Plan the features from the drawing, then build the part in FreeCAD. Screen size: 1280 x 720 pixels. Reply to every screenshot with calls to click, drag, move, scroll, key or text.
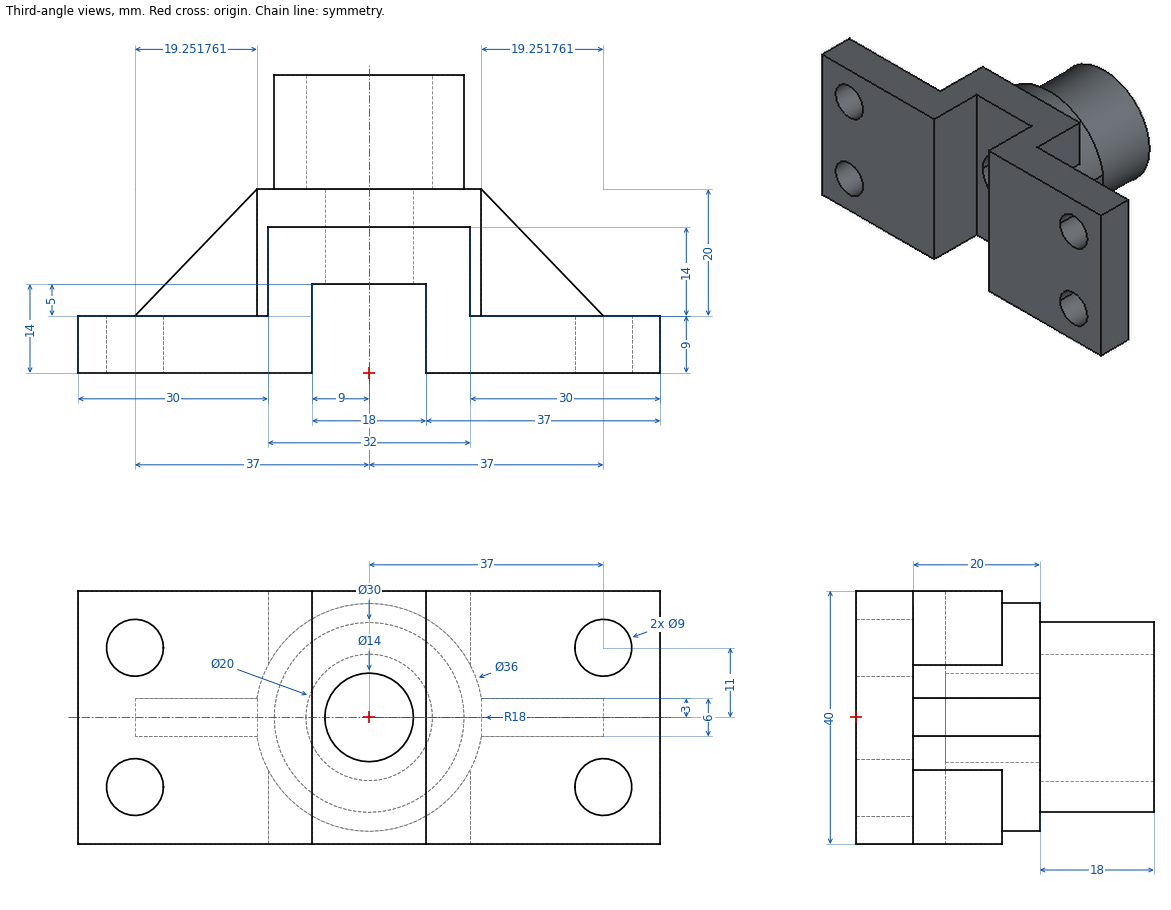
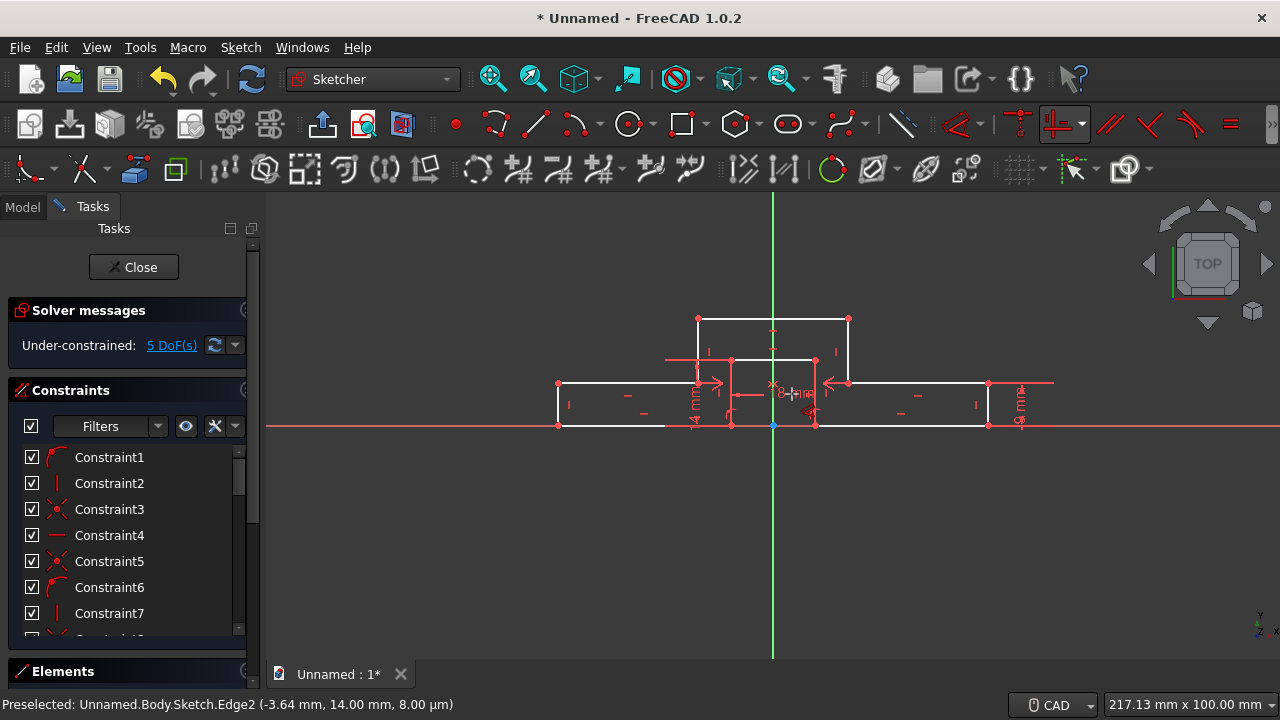
click(867, 426)
click(902, 460)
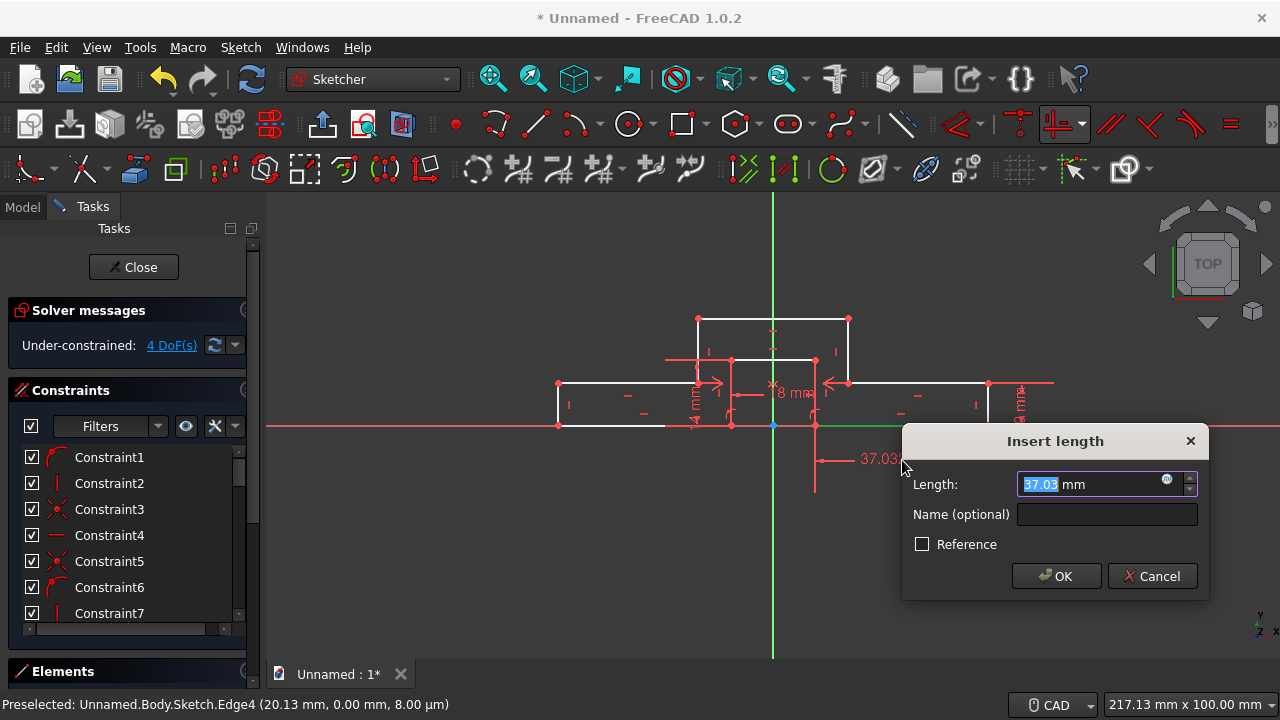
text(37)
key(Return)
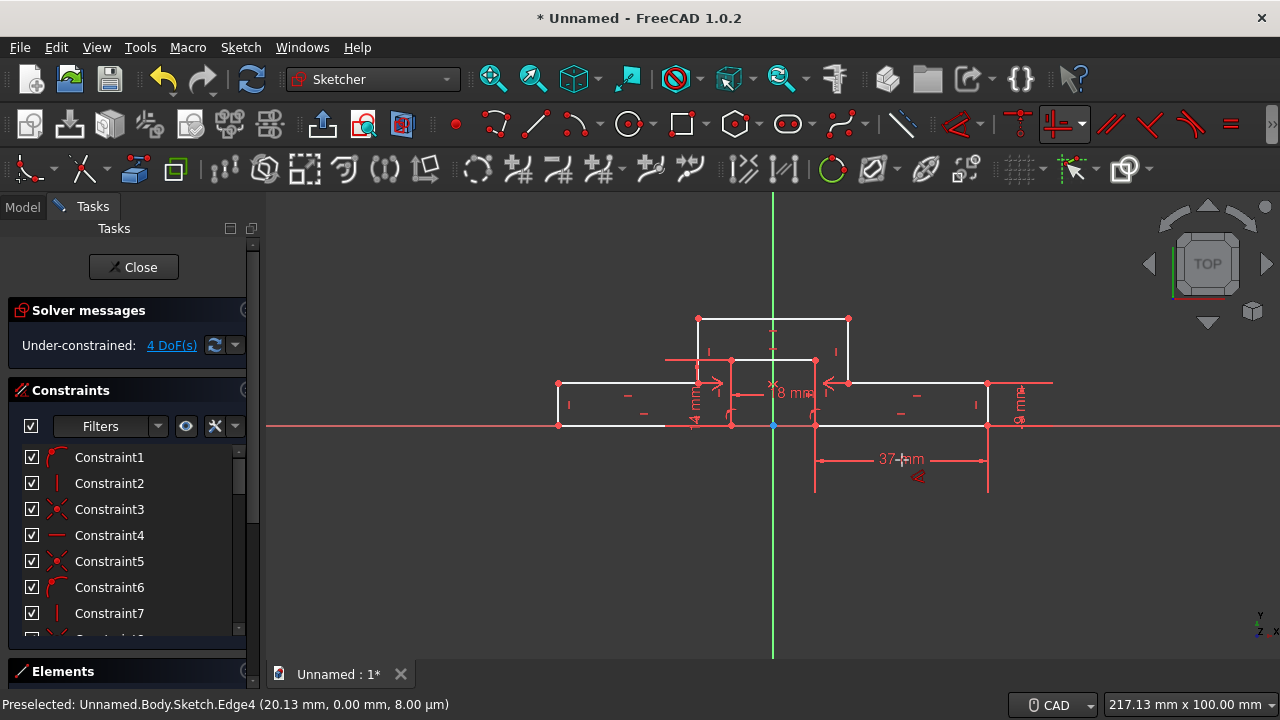
click(946, 383)
click(918, 349)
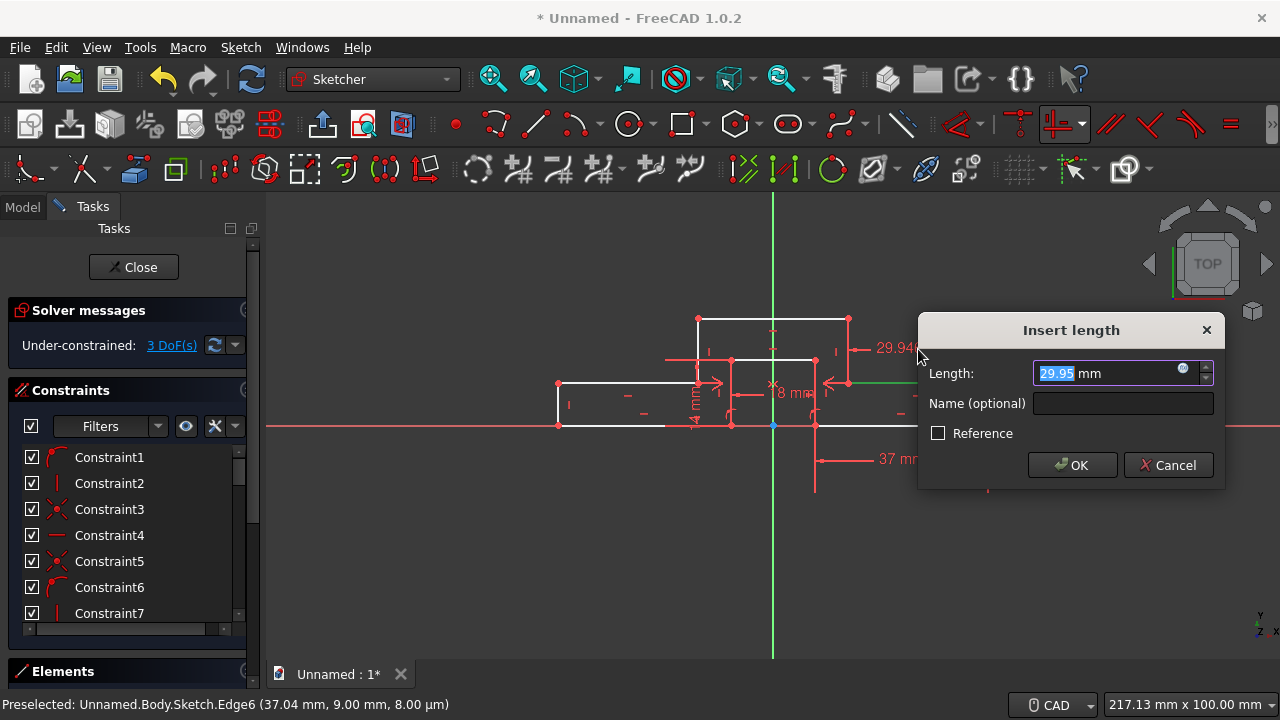
text(30)
key(Return)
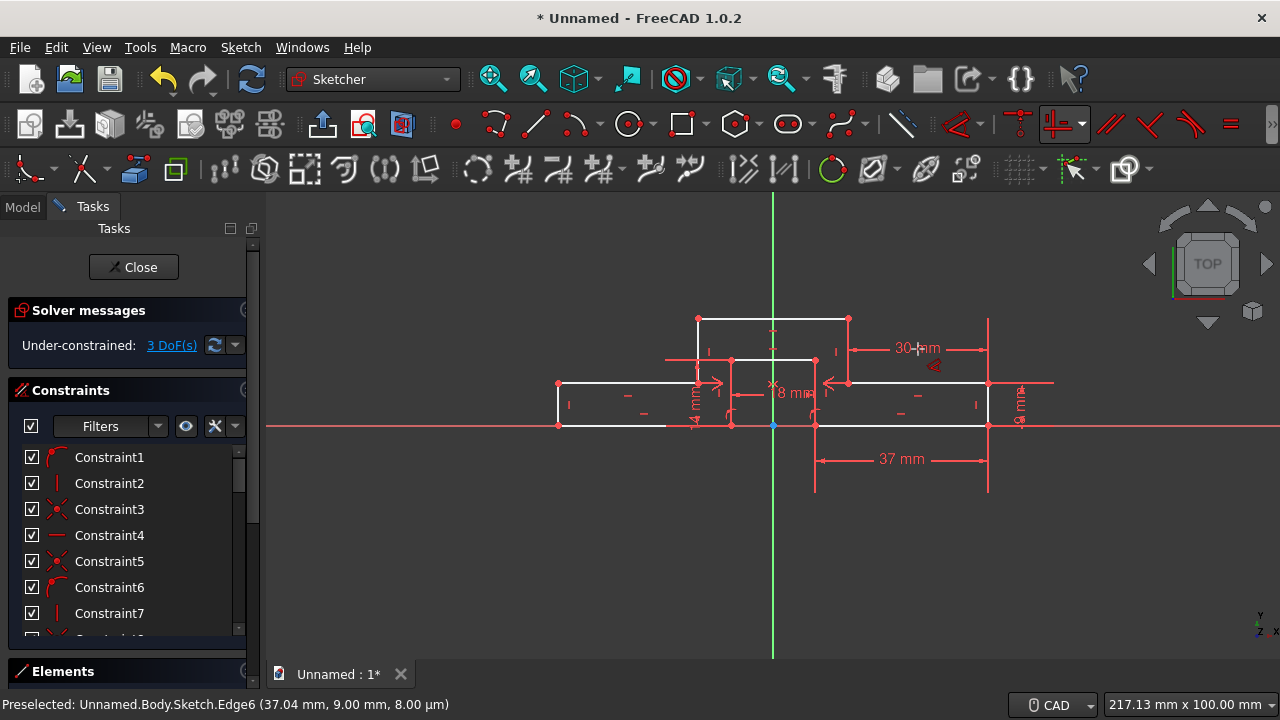
click(848, 364)
click(882, 329)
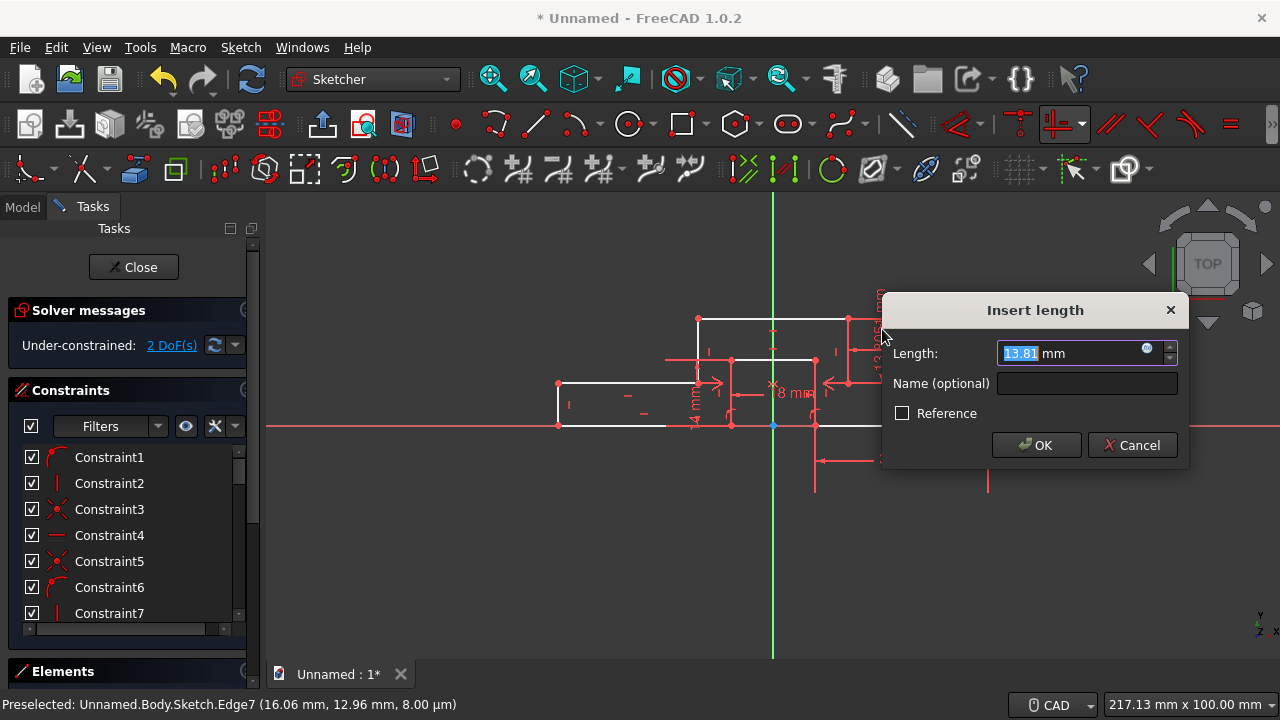
text(14)
key(Return)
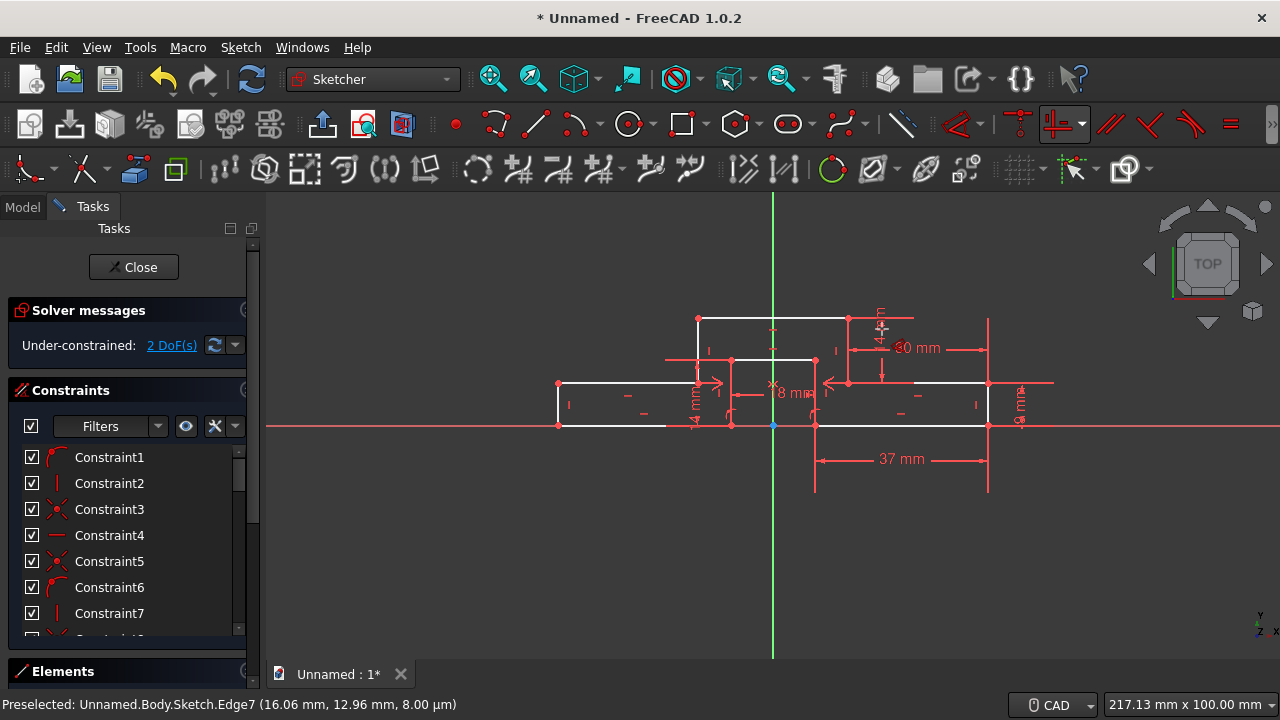
click(803, 318)
click(739, 284)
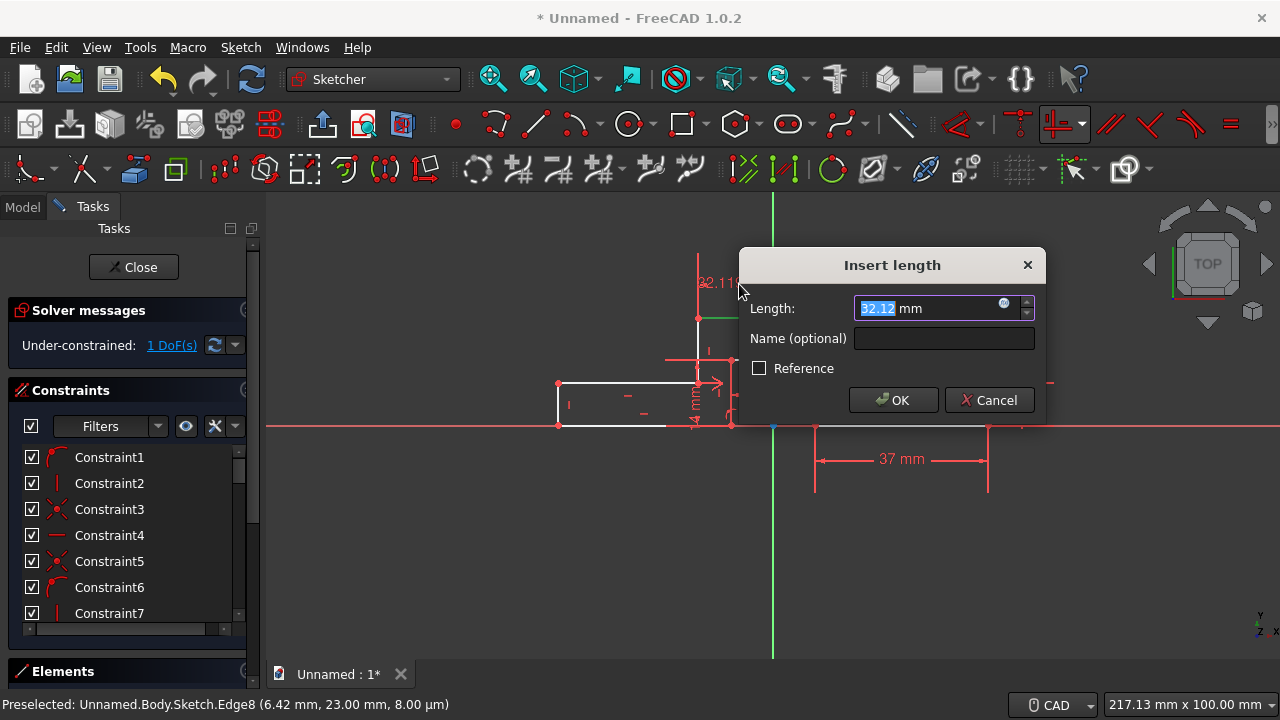
text(32)
key(Return)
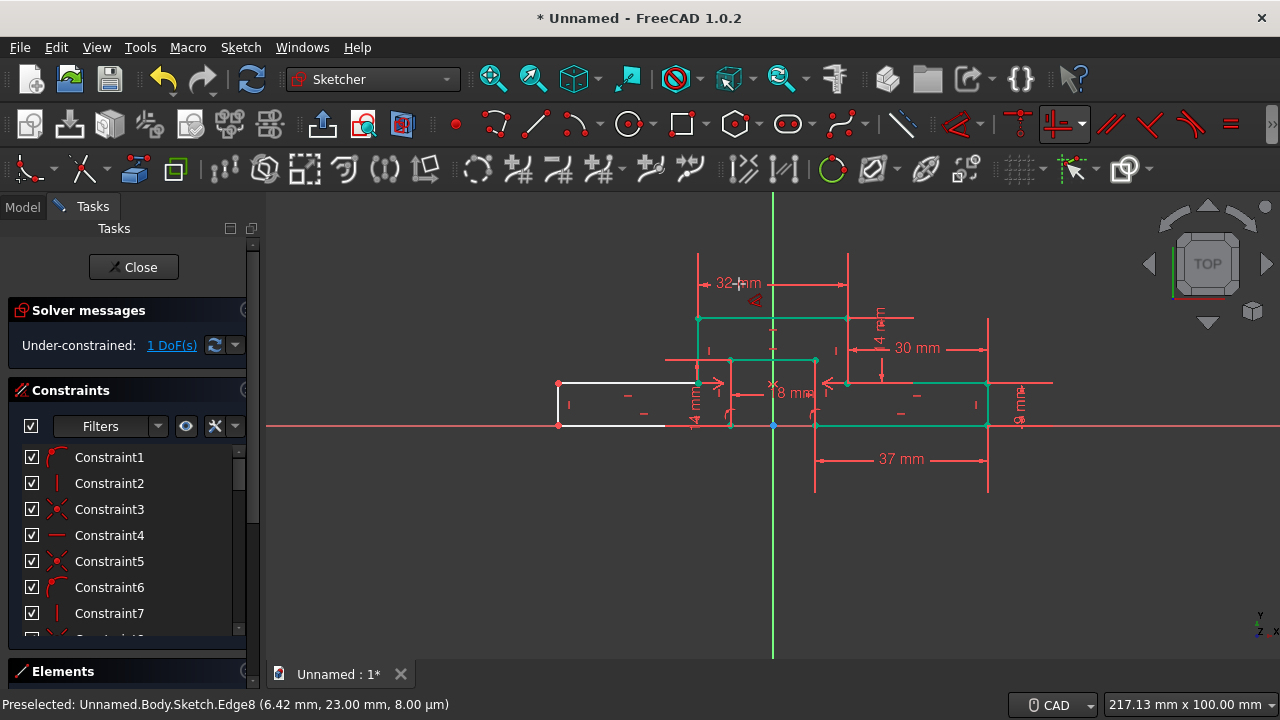
click(656, 383)
click(628, 349)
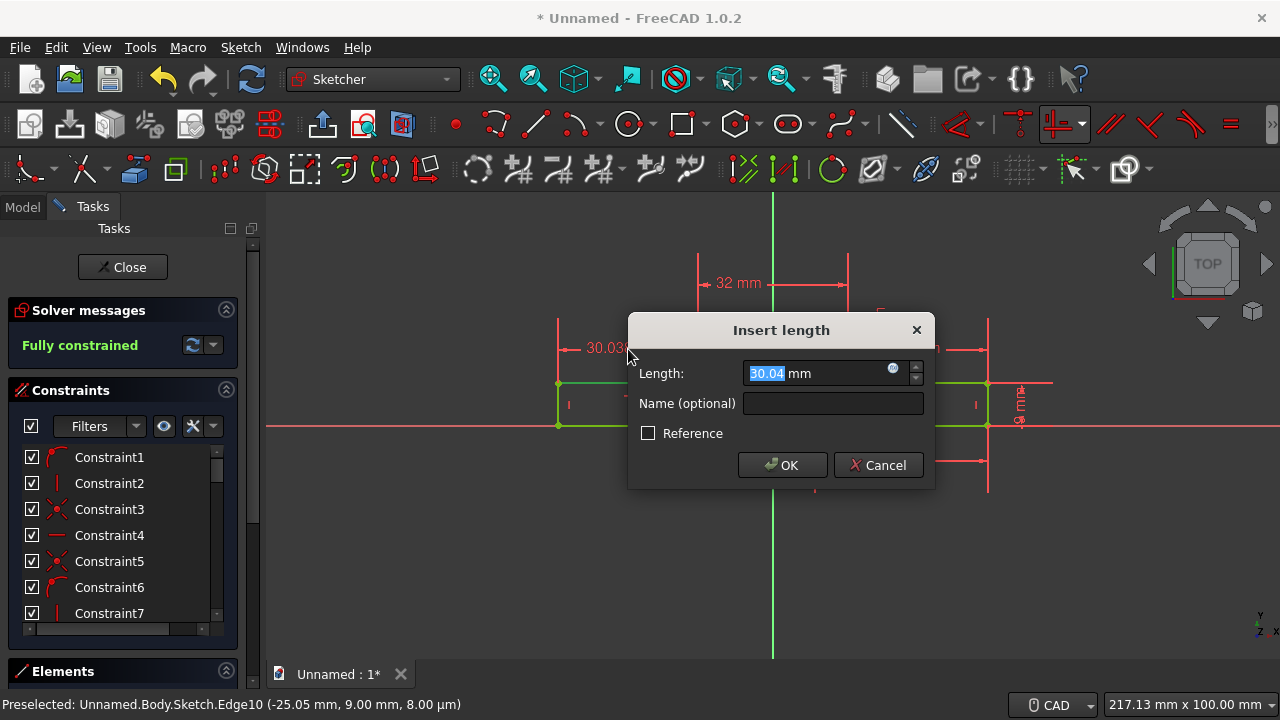
text(30)
key(Return)
key(Escape)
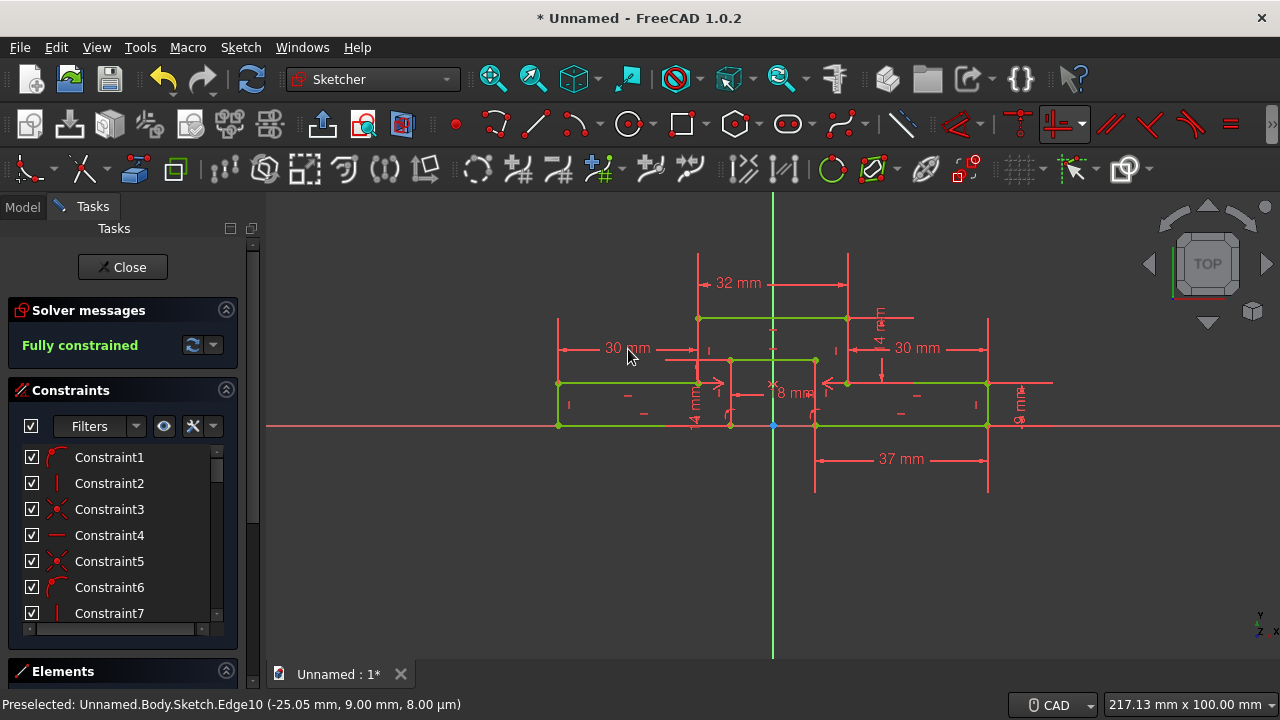
click(123, 267)